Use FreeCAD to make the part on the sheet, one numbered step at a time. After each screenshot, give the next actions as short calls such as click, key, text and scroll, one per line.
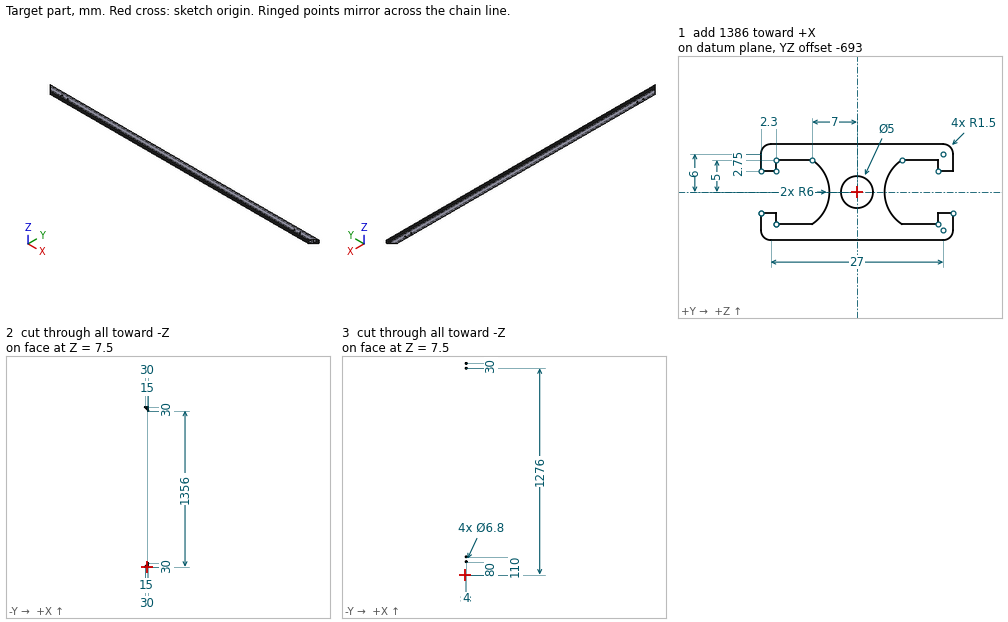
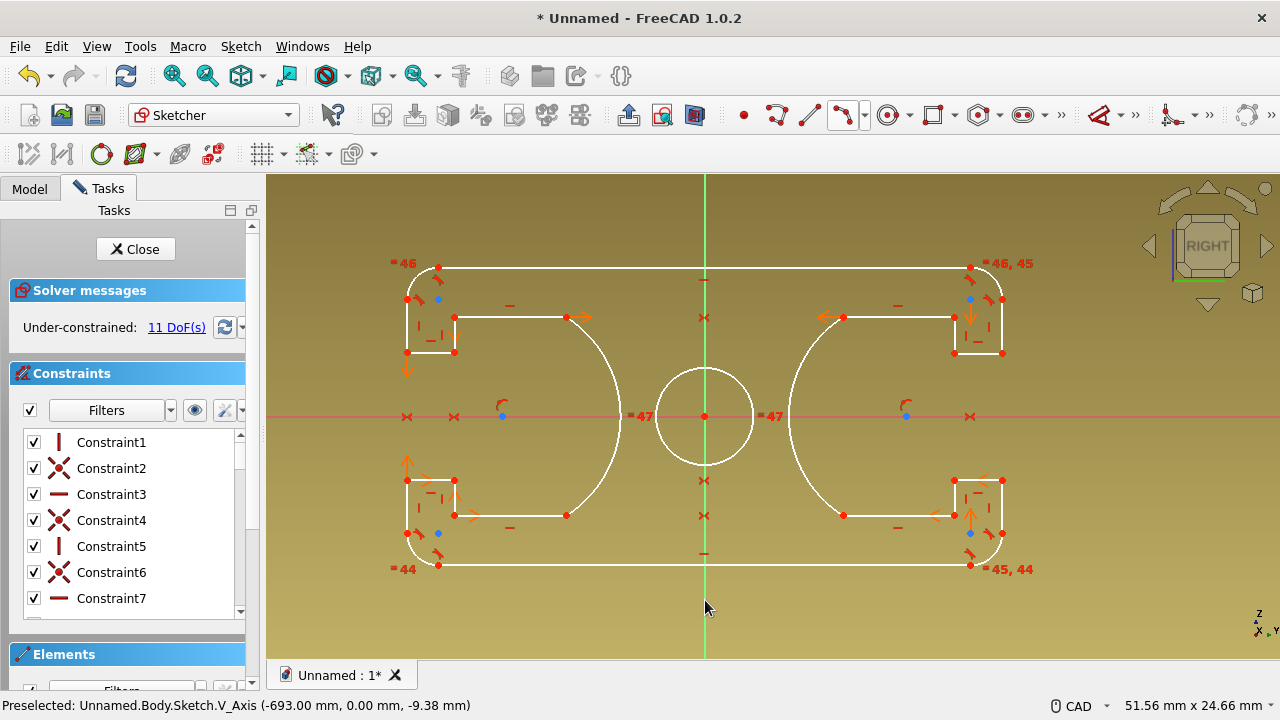
click(455, 353)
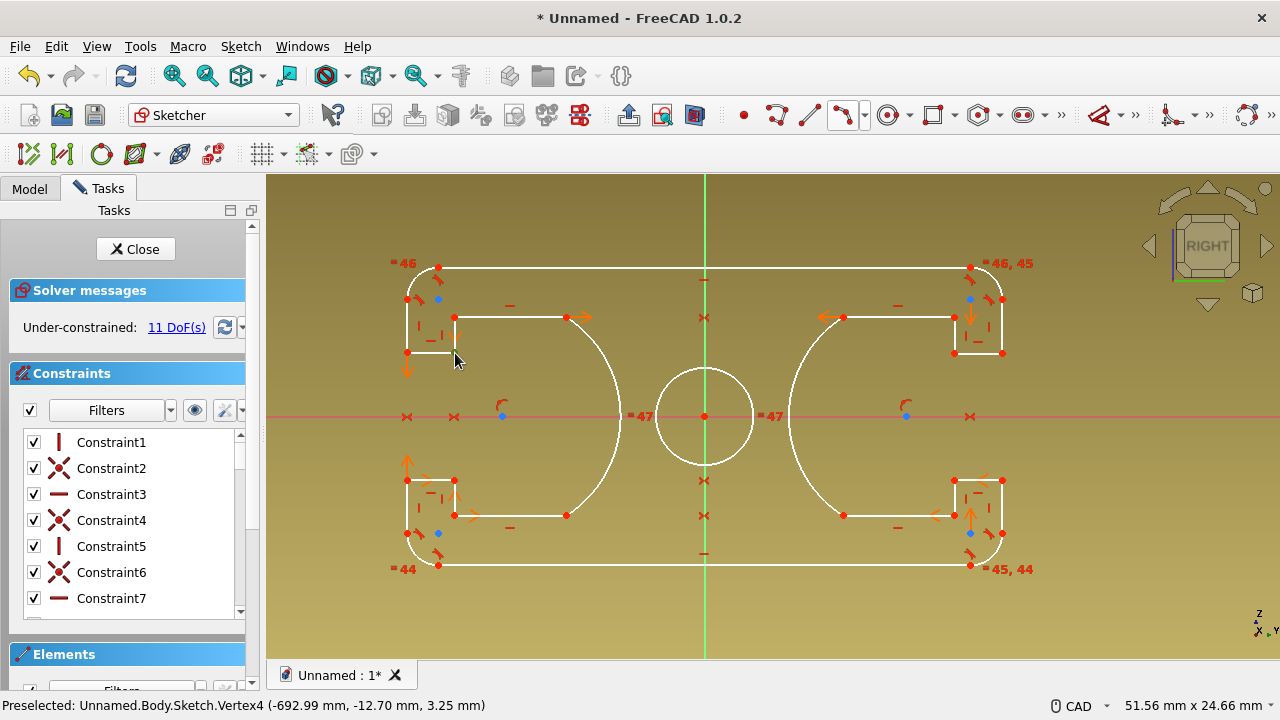
click(955, 354)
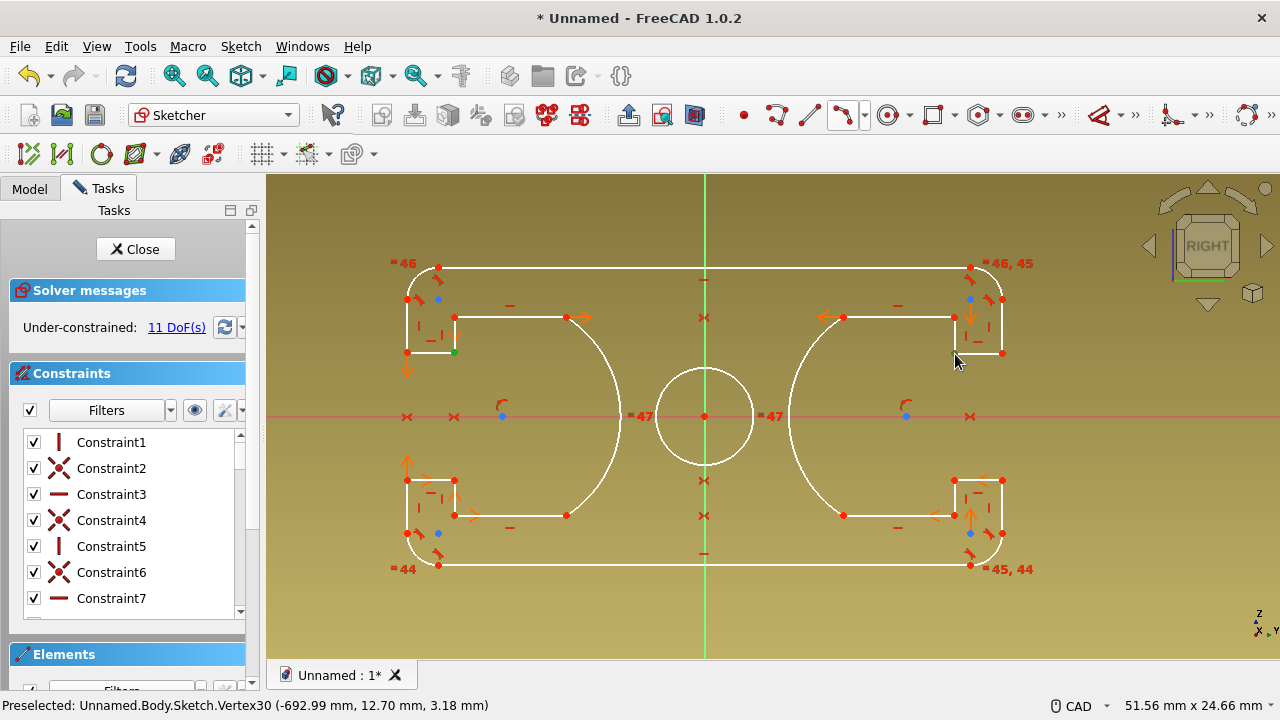
click(705, 600)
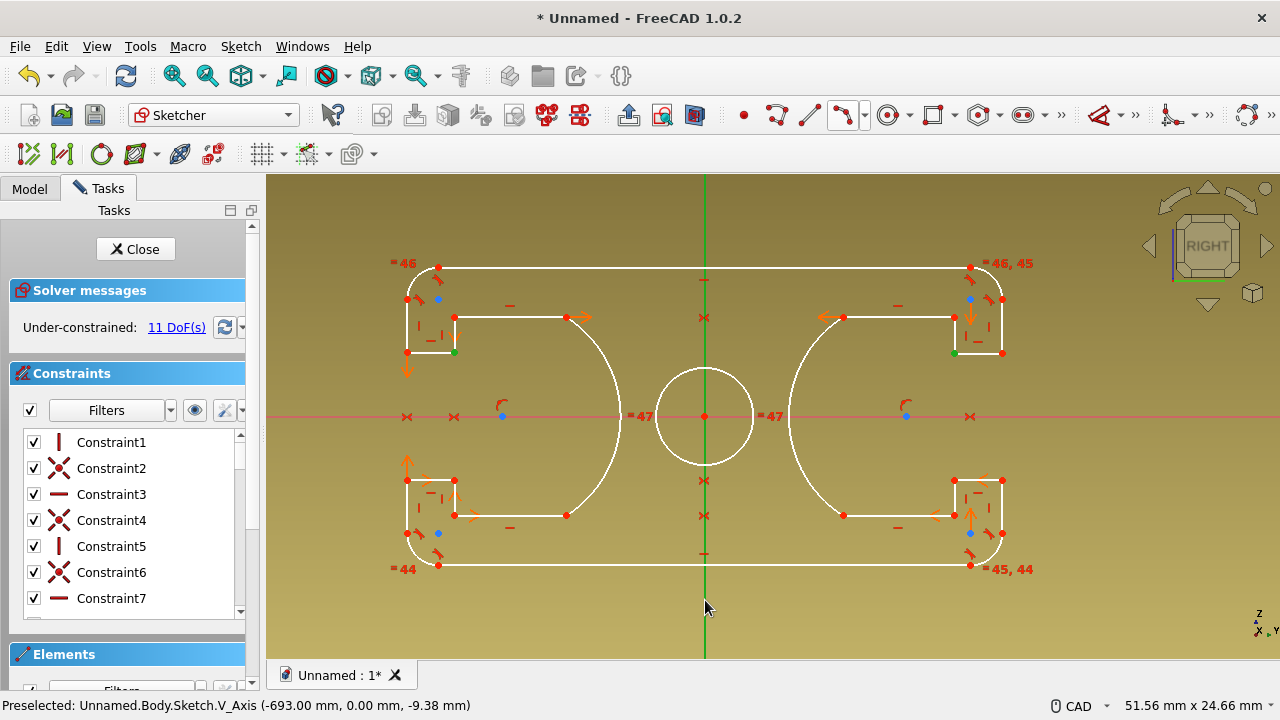
key(s)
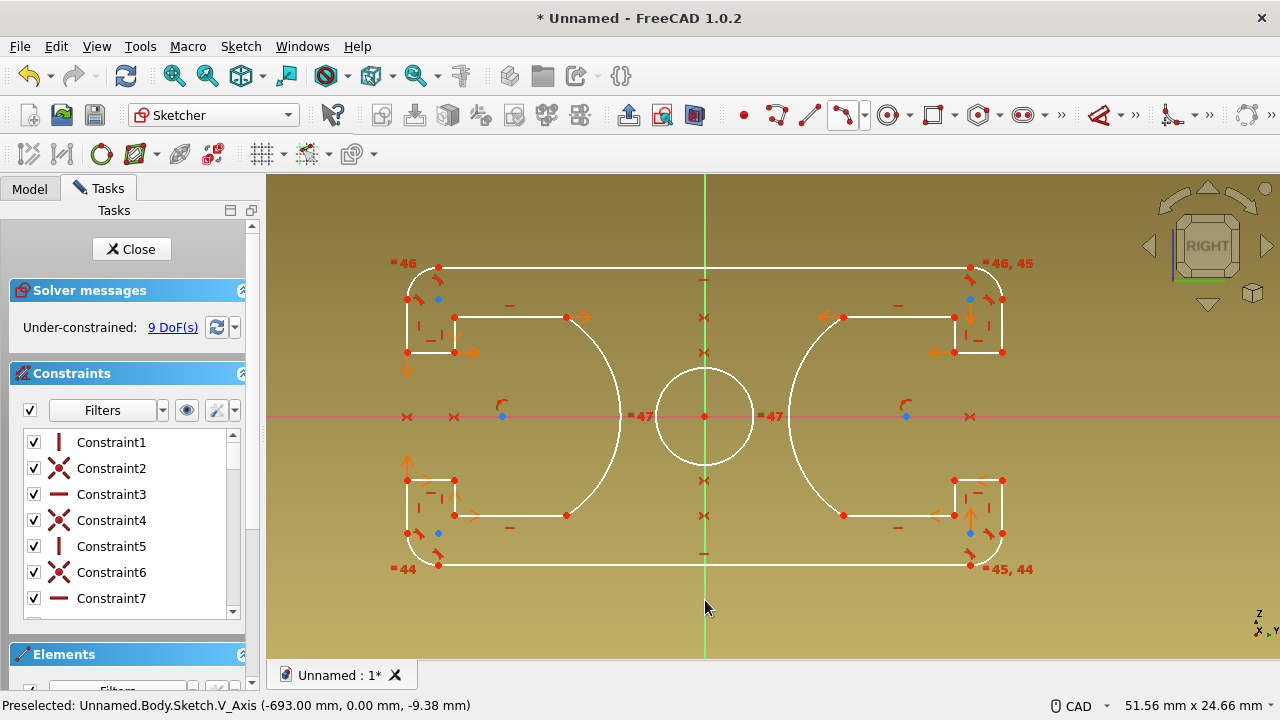
click(611, 462)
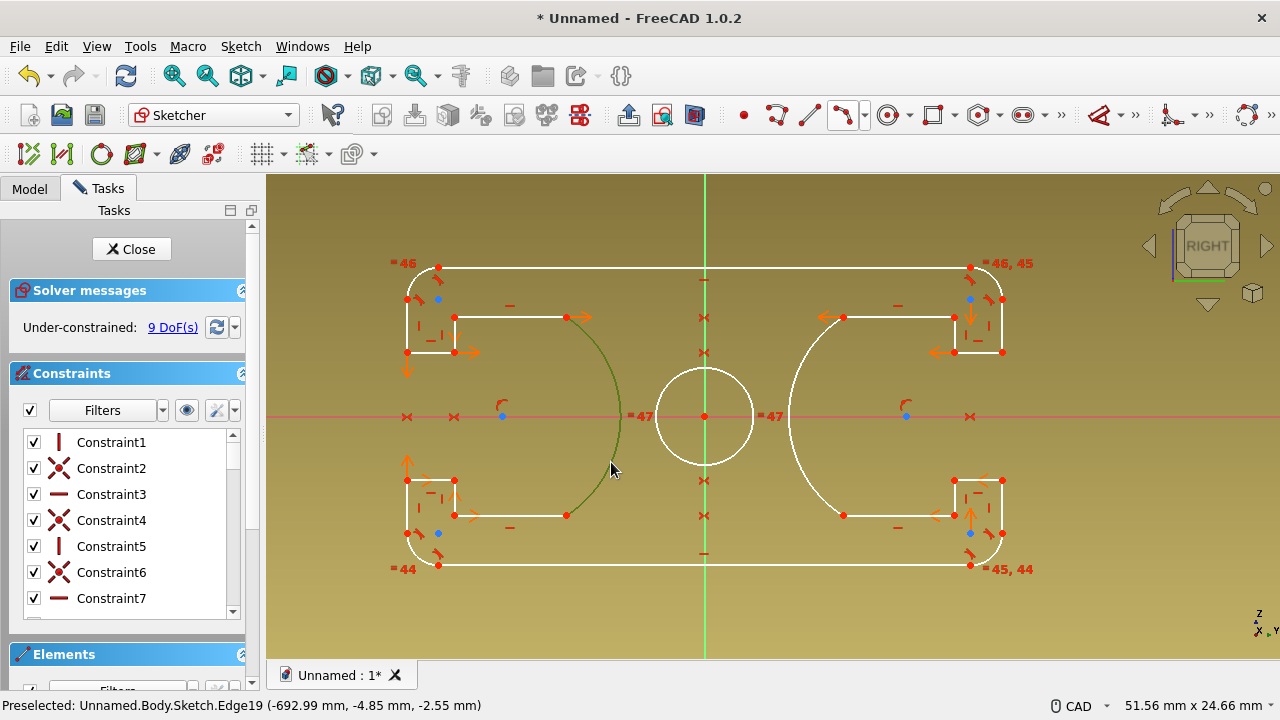
key(k)
key(r)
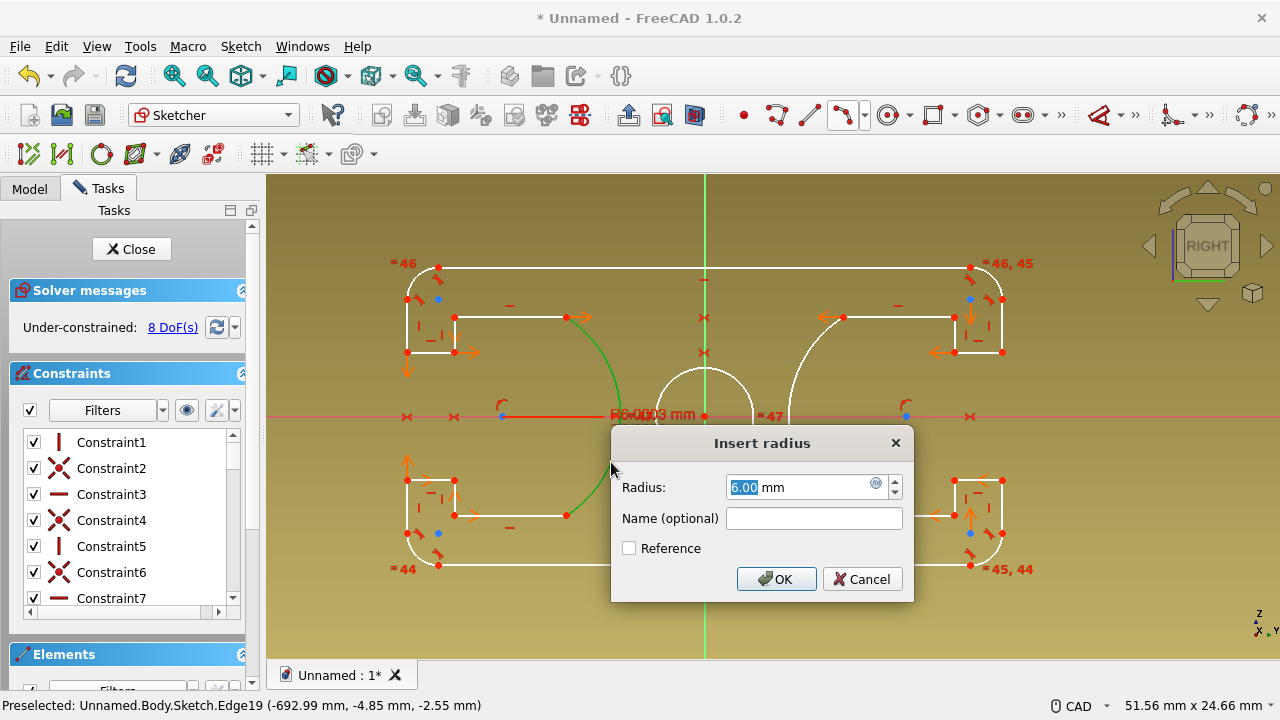
text(6)
key(Return)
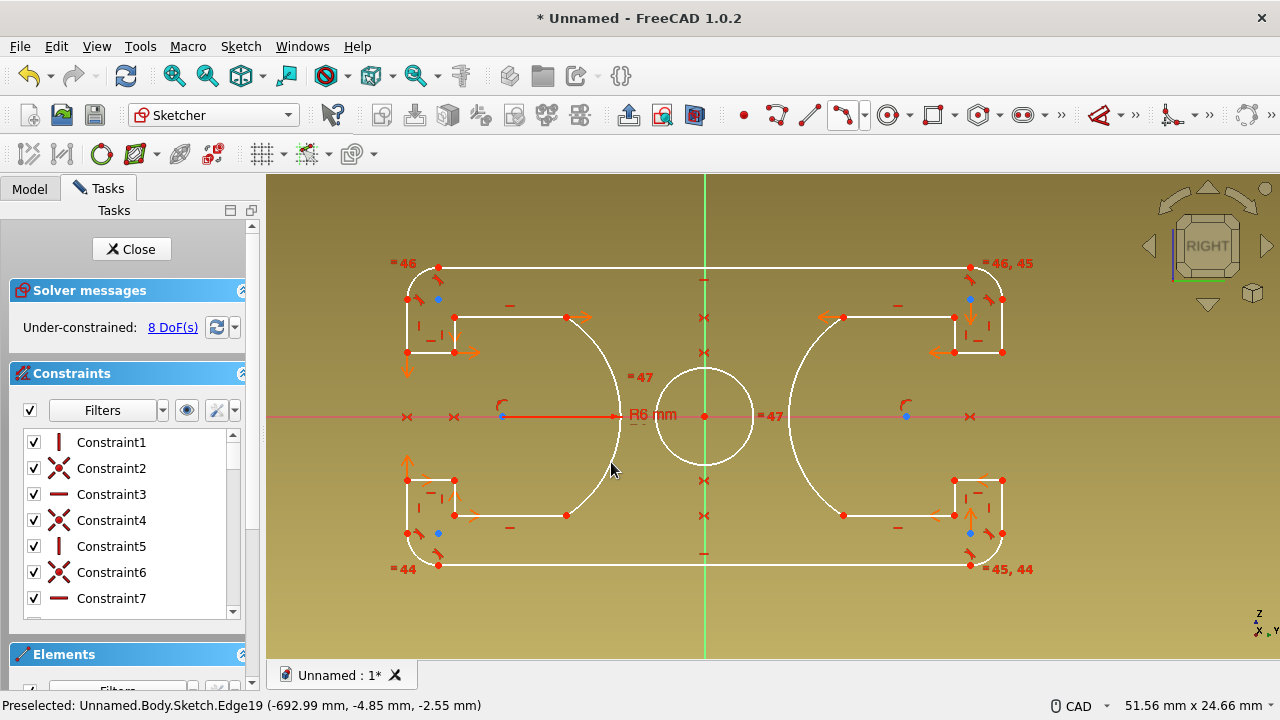
scroll(411, 548, up, 2)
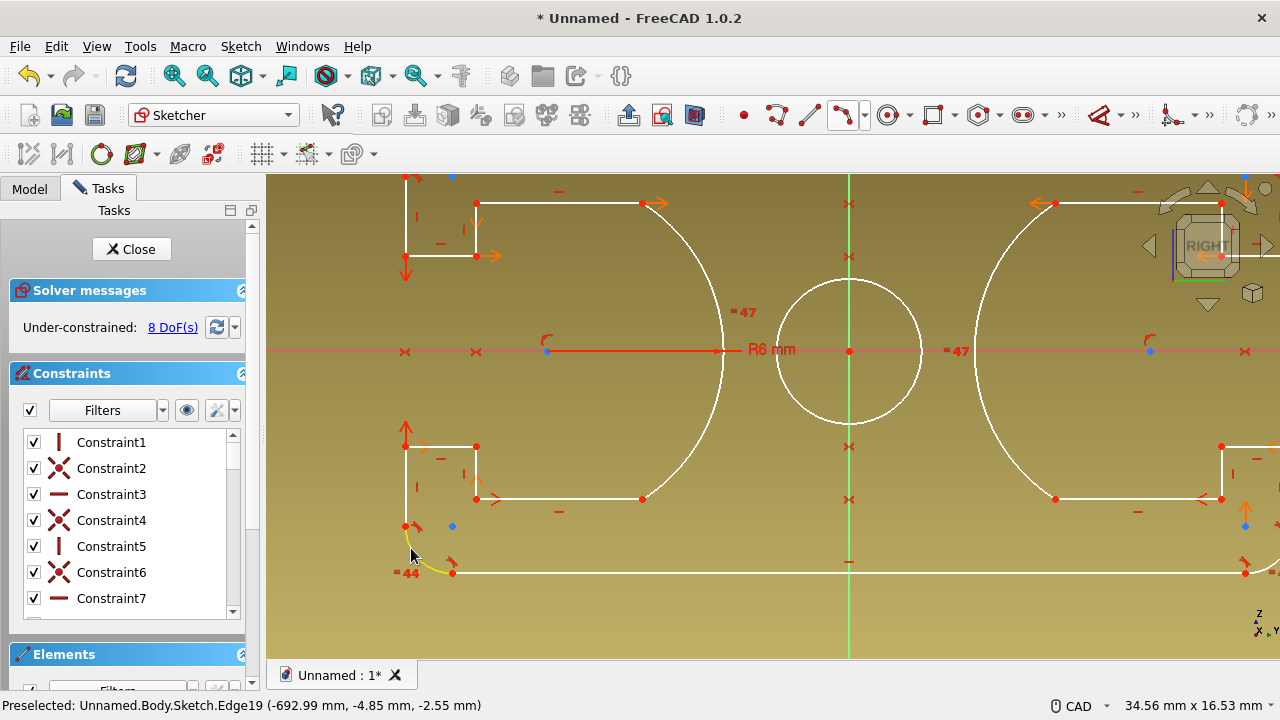
click(411, 548)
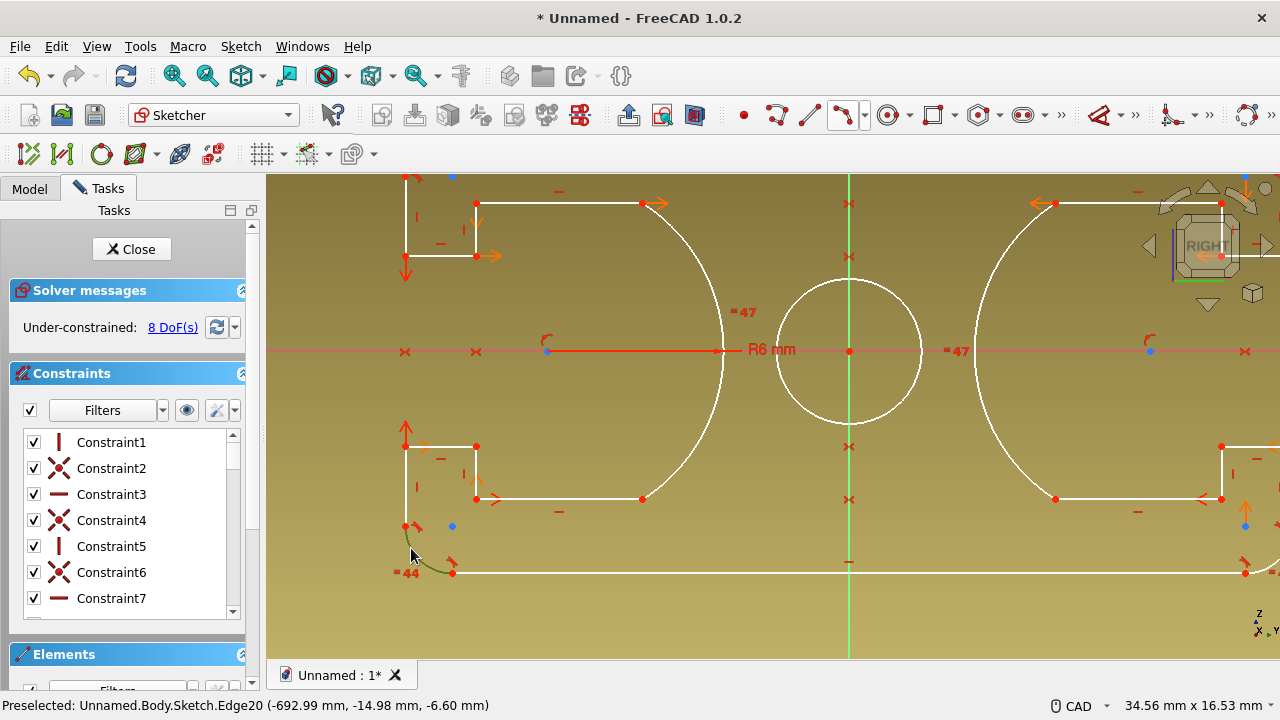
click(1120, 116)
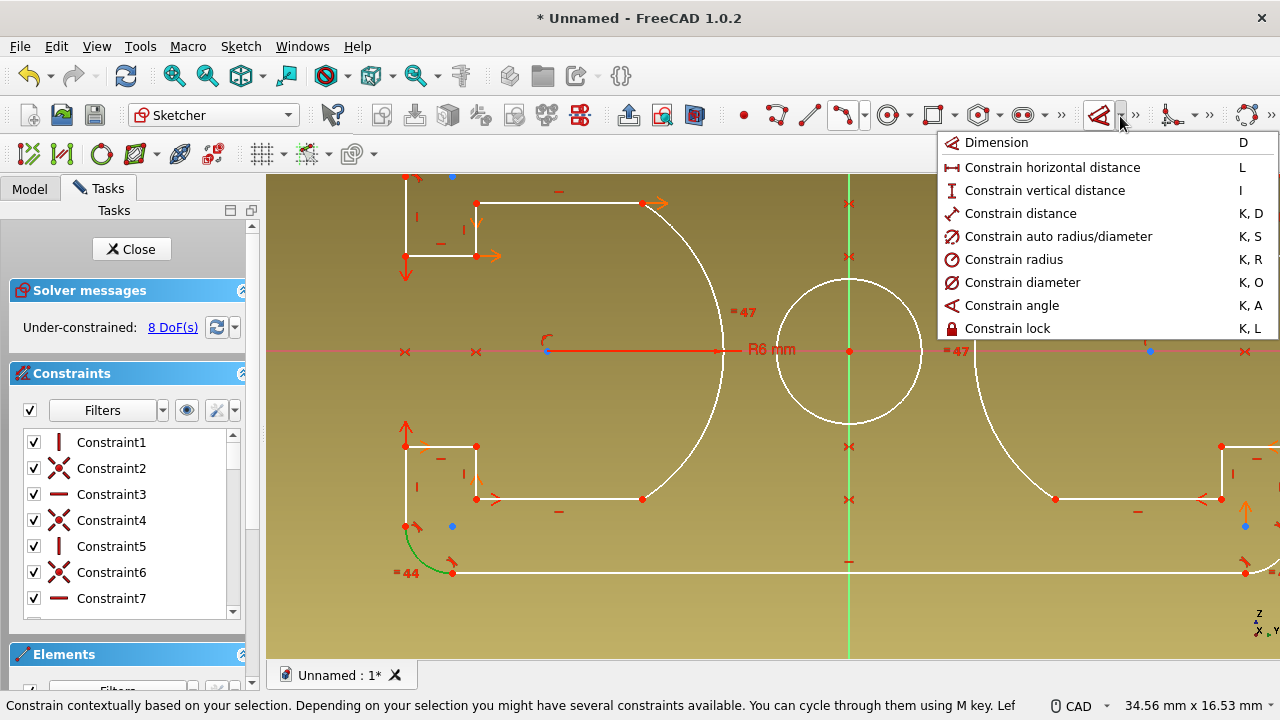
click(1108, 260)